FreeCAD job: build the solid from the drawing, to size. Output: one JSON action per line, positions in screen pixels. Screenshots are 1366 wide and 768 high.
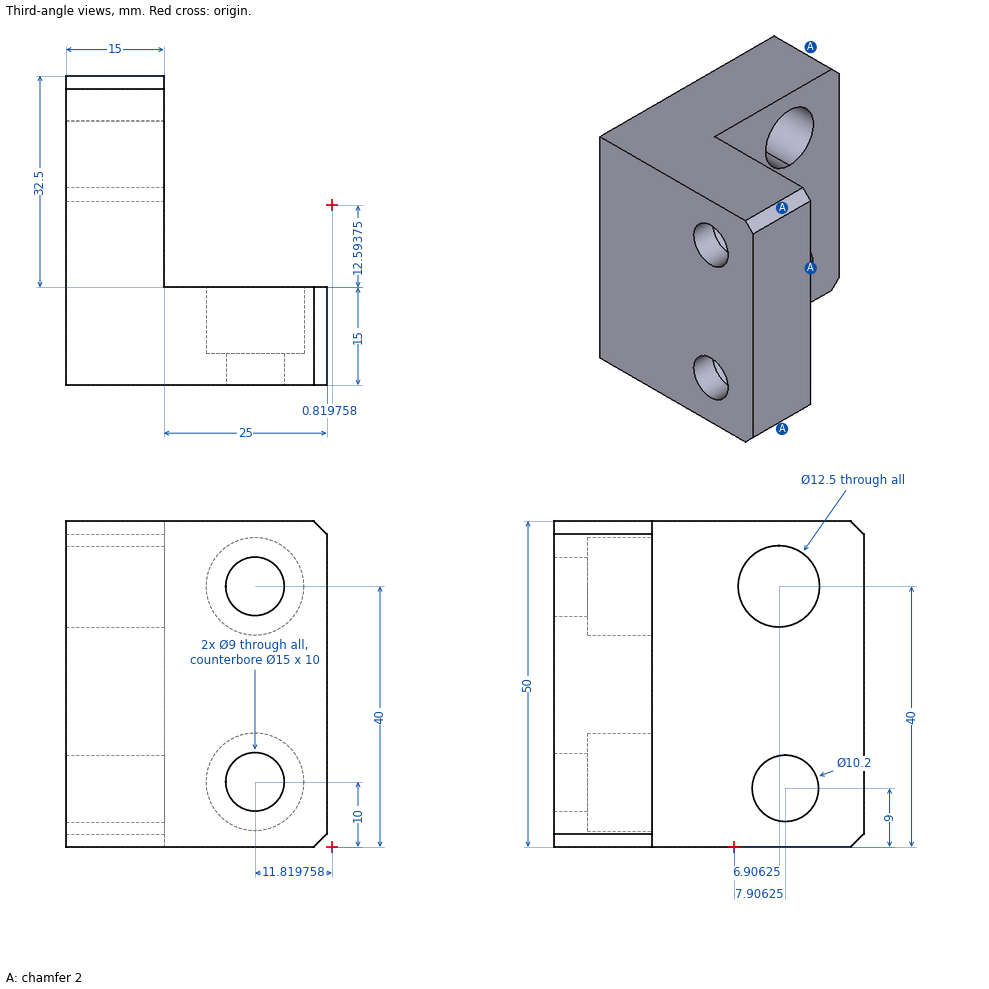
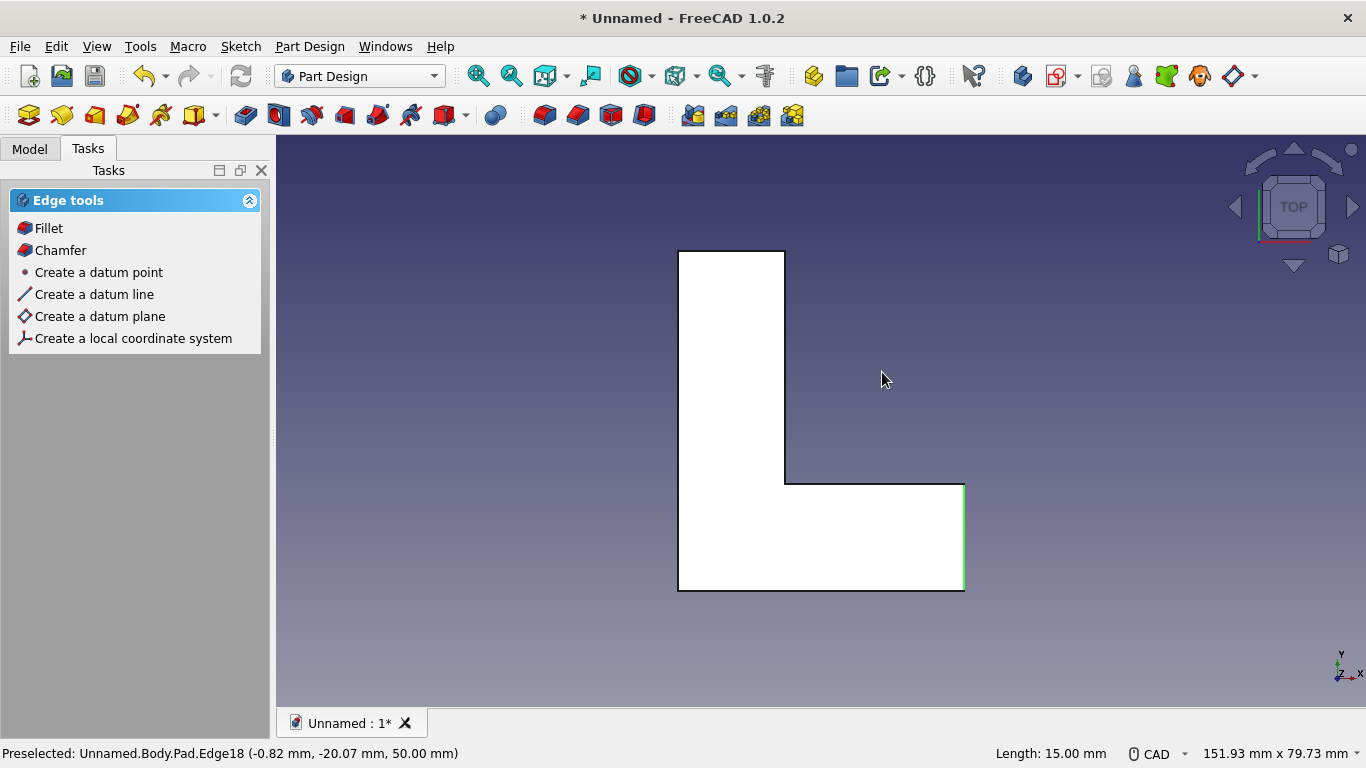
{"action": "left_click", "coordinate": [731, 250], "text": "ctrl"}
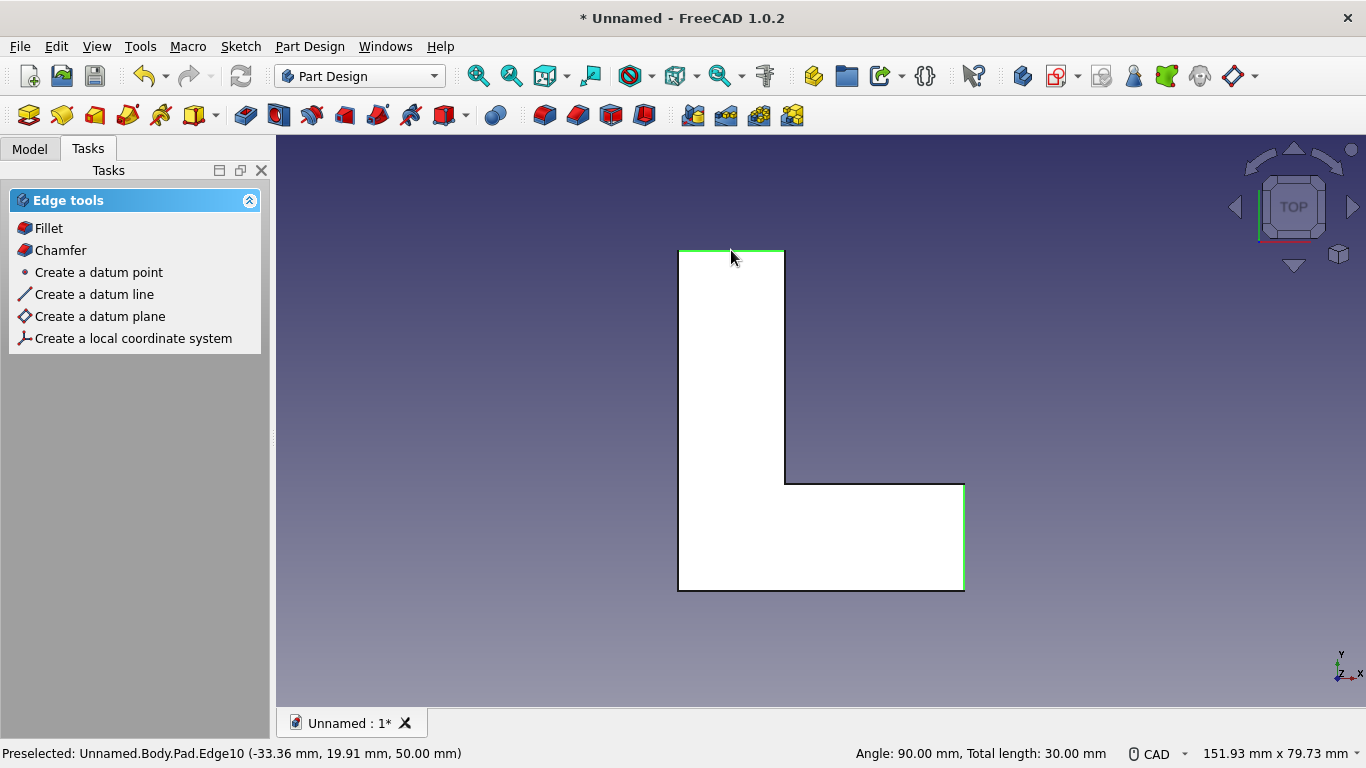
{"action": "key", "text": "1"}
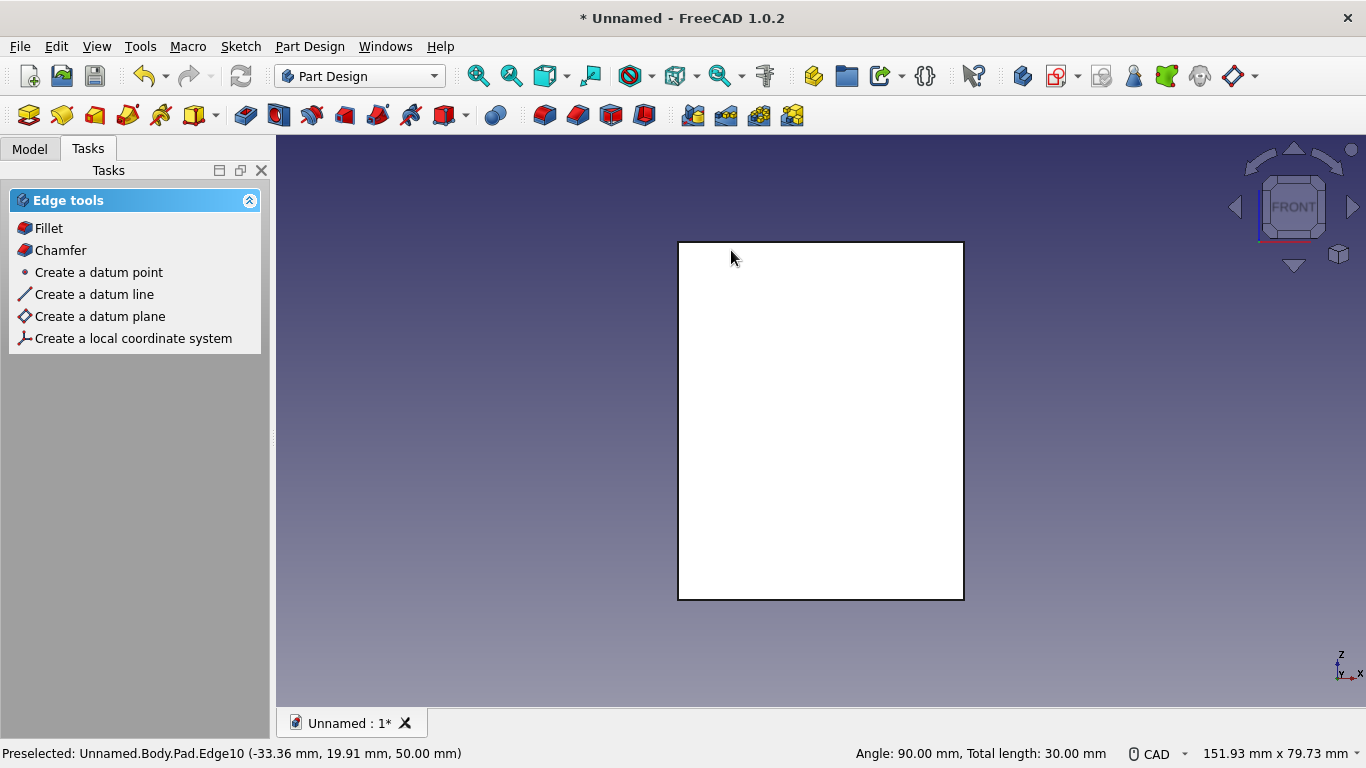
{"action": "key", "text": "3"}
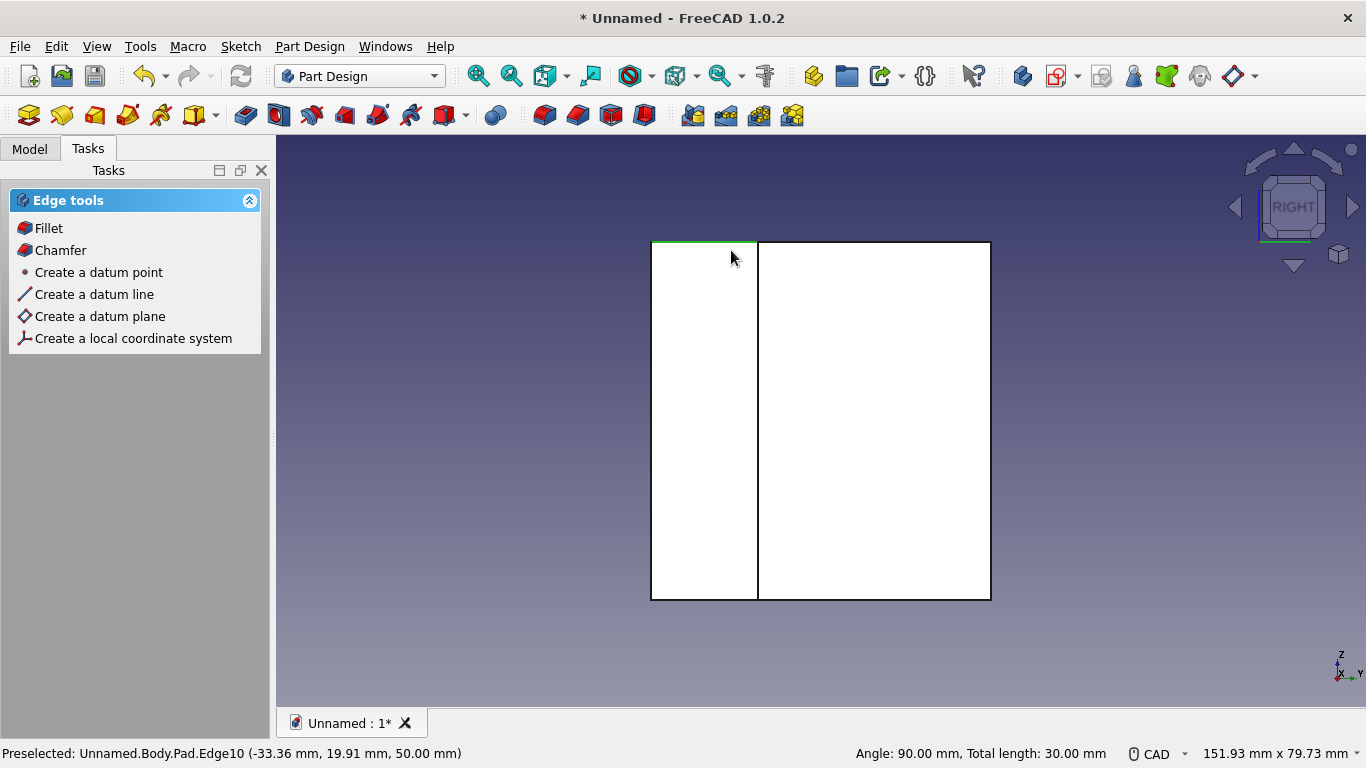
{"action": "left_click", "coordinate": [704, 599], "text": "ctrl"}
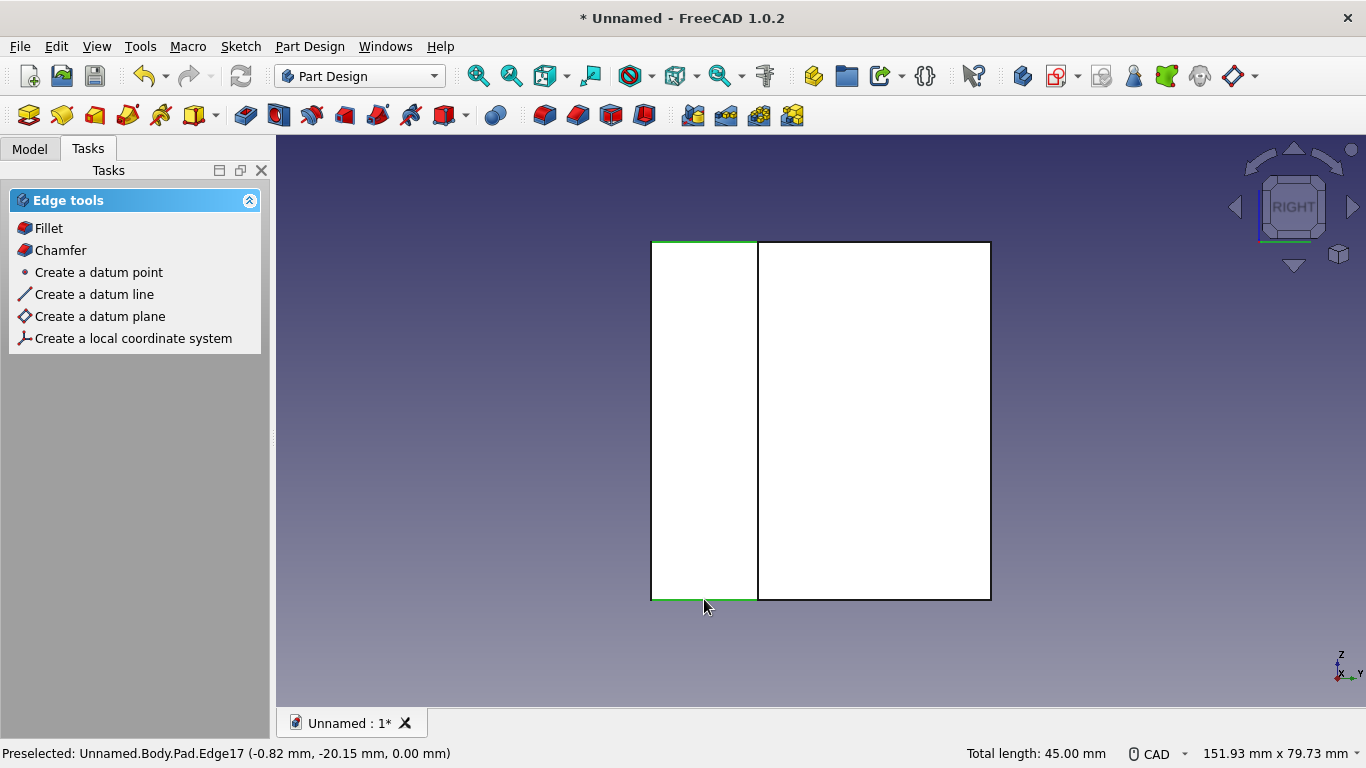
{"action": "key", "text": "5"}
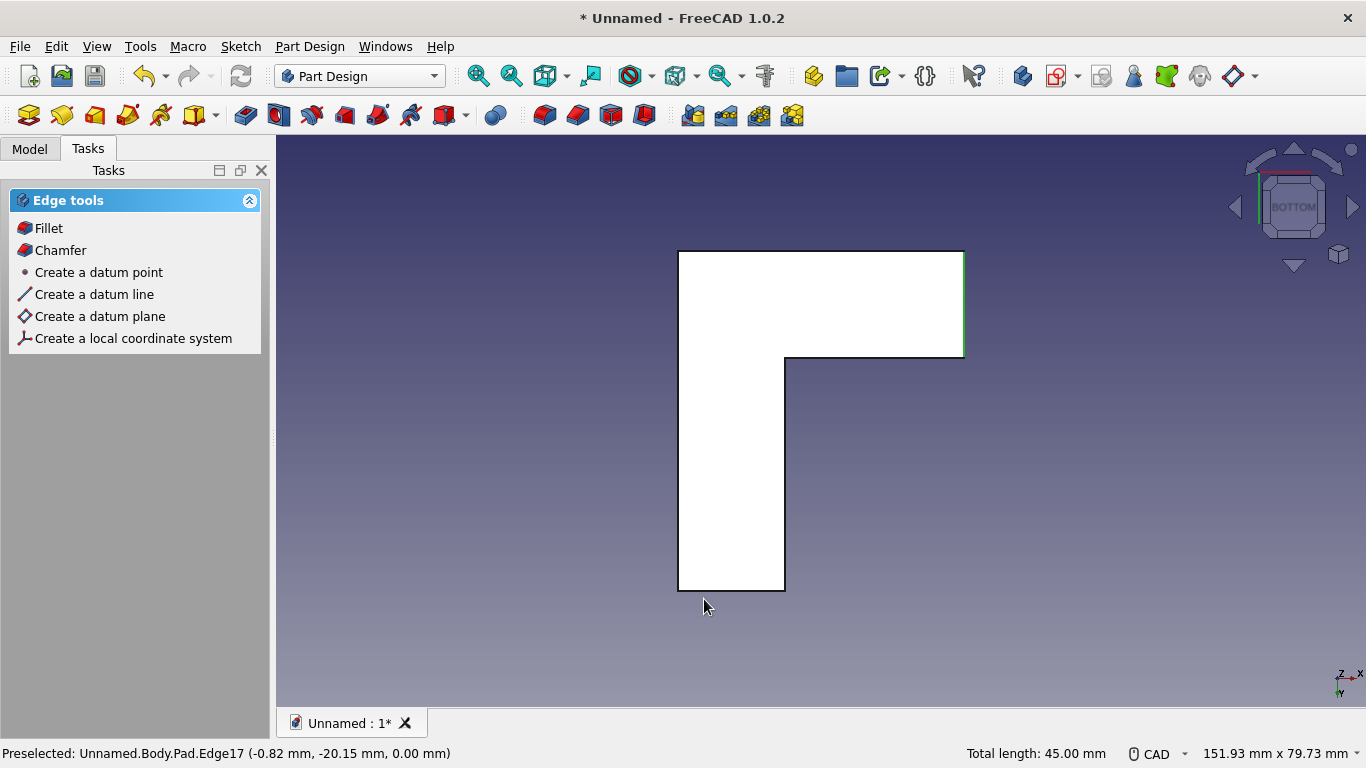
{"action": "left_click", "coordinate": [731, 590], "text": "ctrl"}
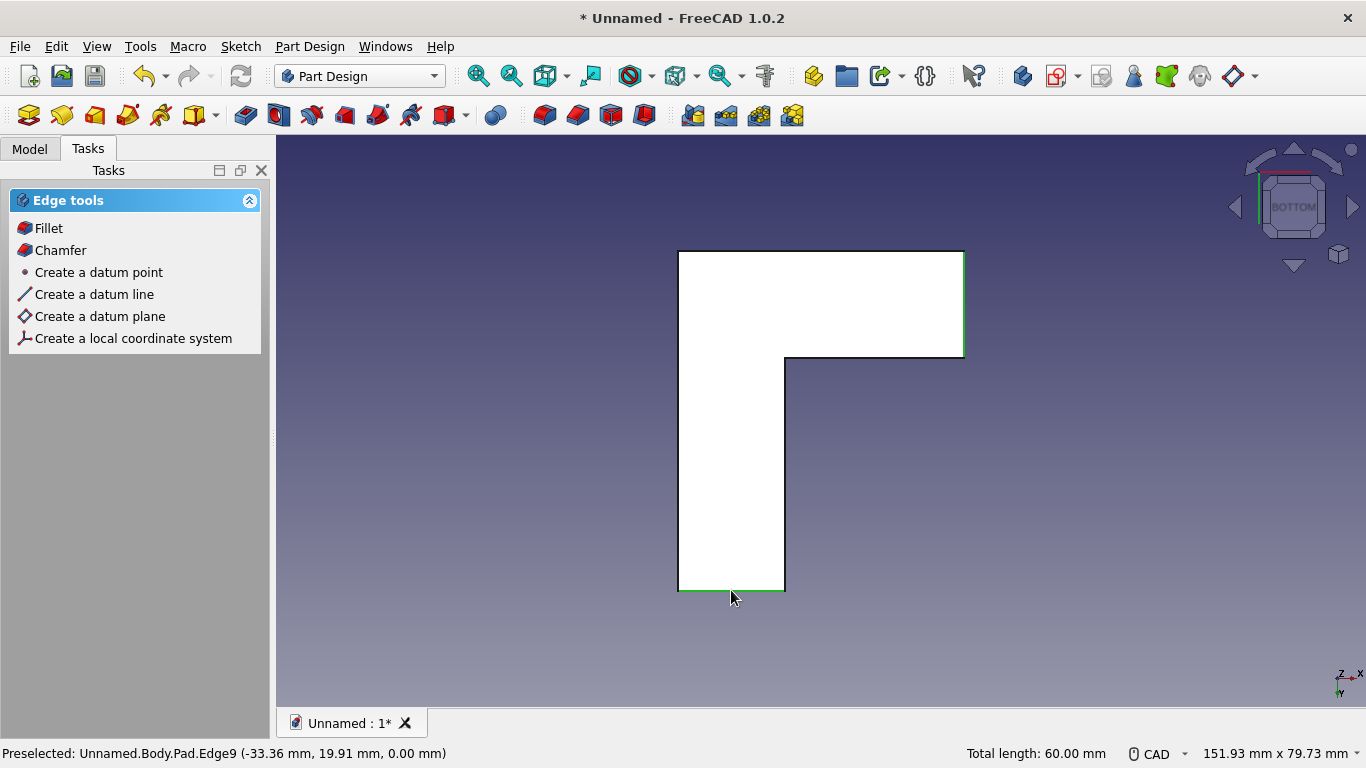
{"action": "left_click", "coordinate": [578, 116]}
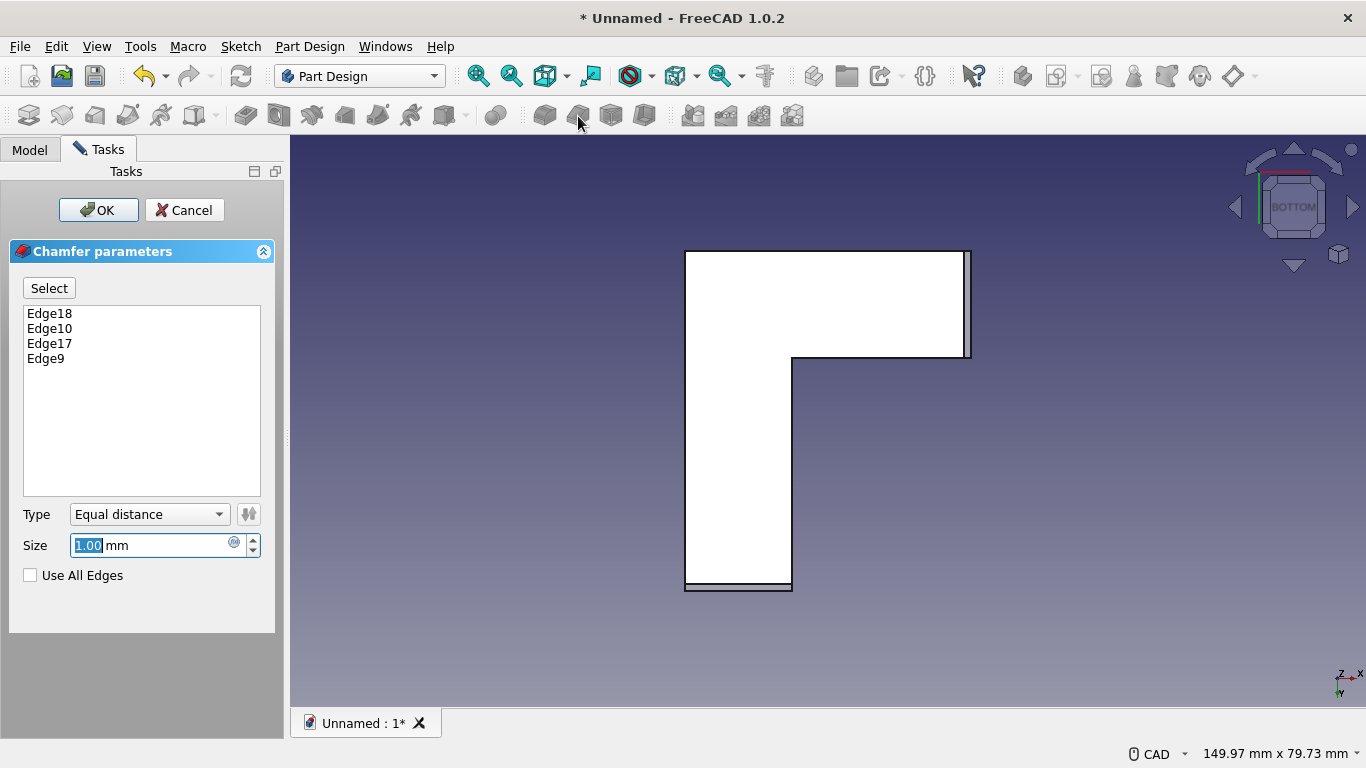
{"action": "type", "text": "2"}
{"action": "key", "text": "Tab"}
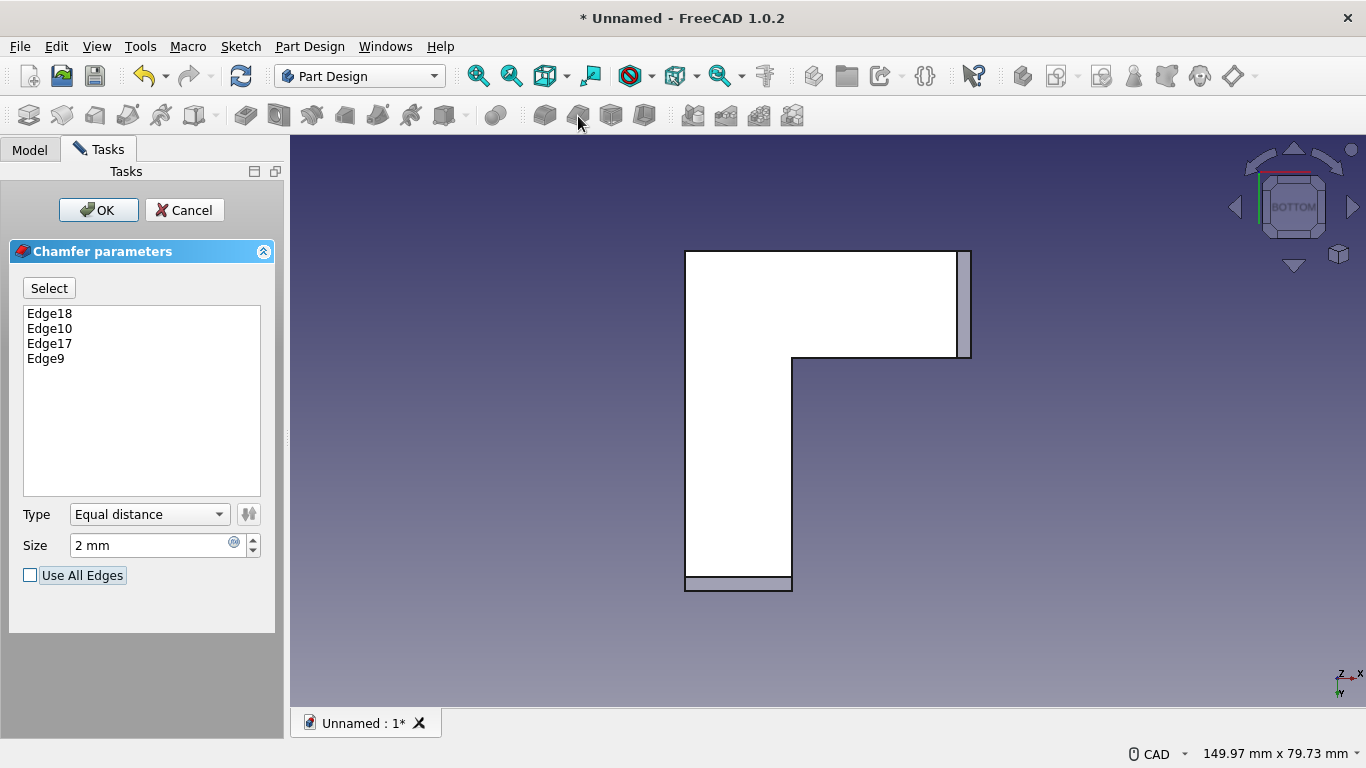
{"action": "left_click", "coordinate": [99, 210]}